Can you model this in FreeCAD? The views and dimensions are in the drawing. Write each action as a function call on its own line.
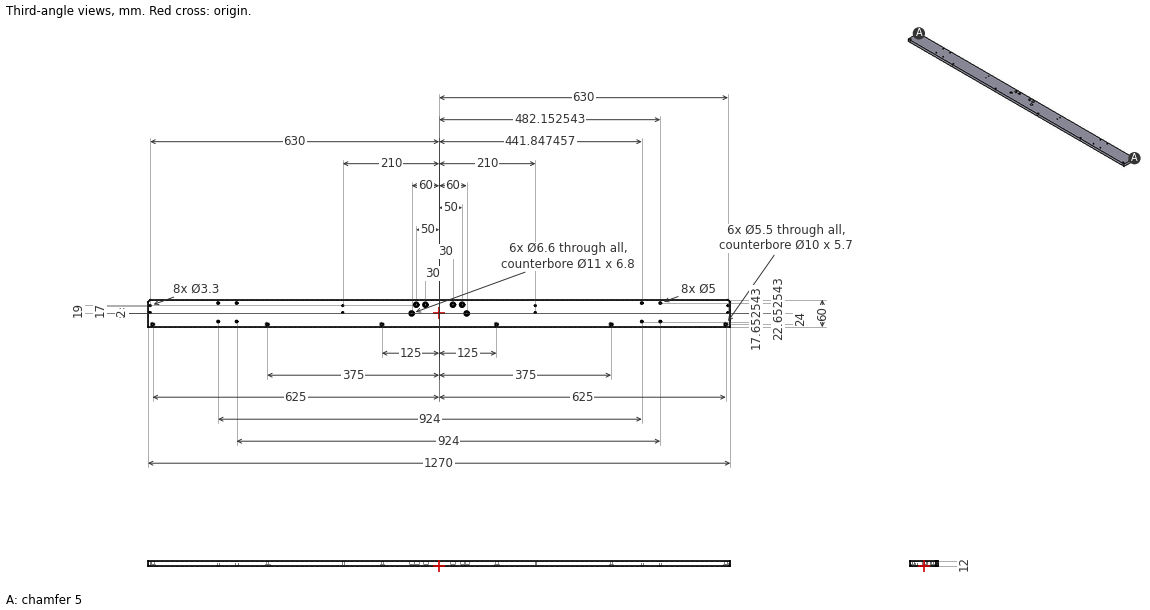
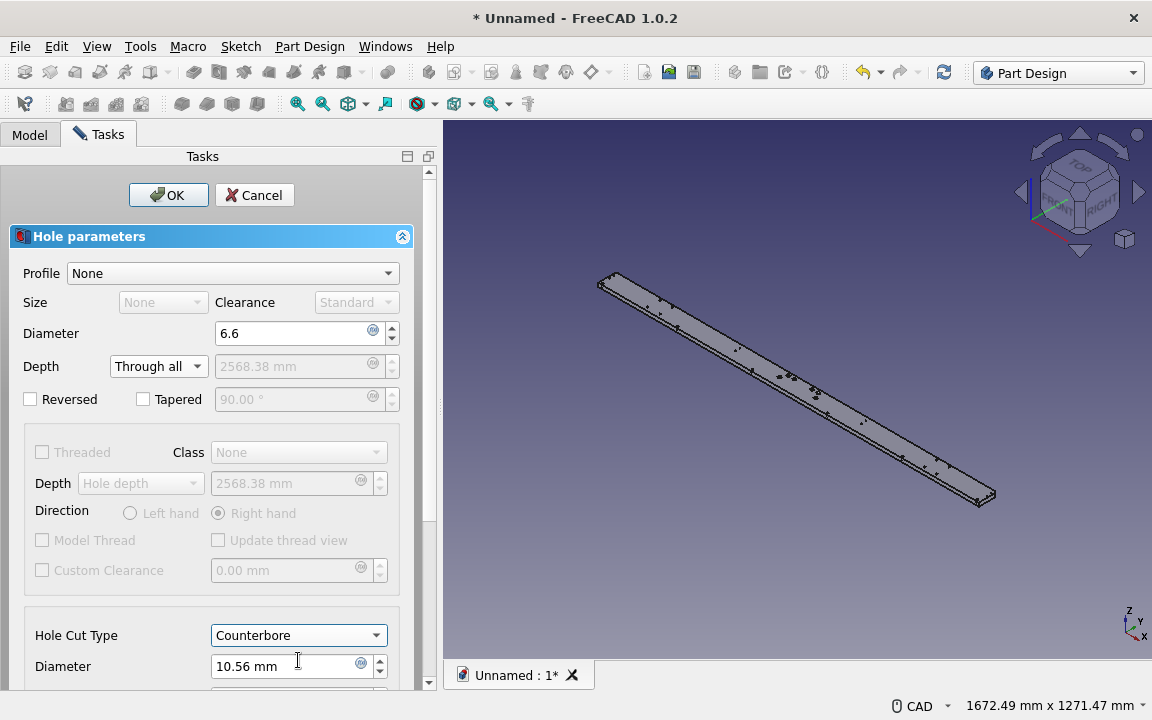
triple_click(292, 666)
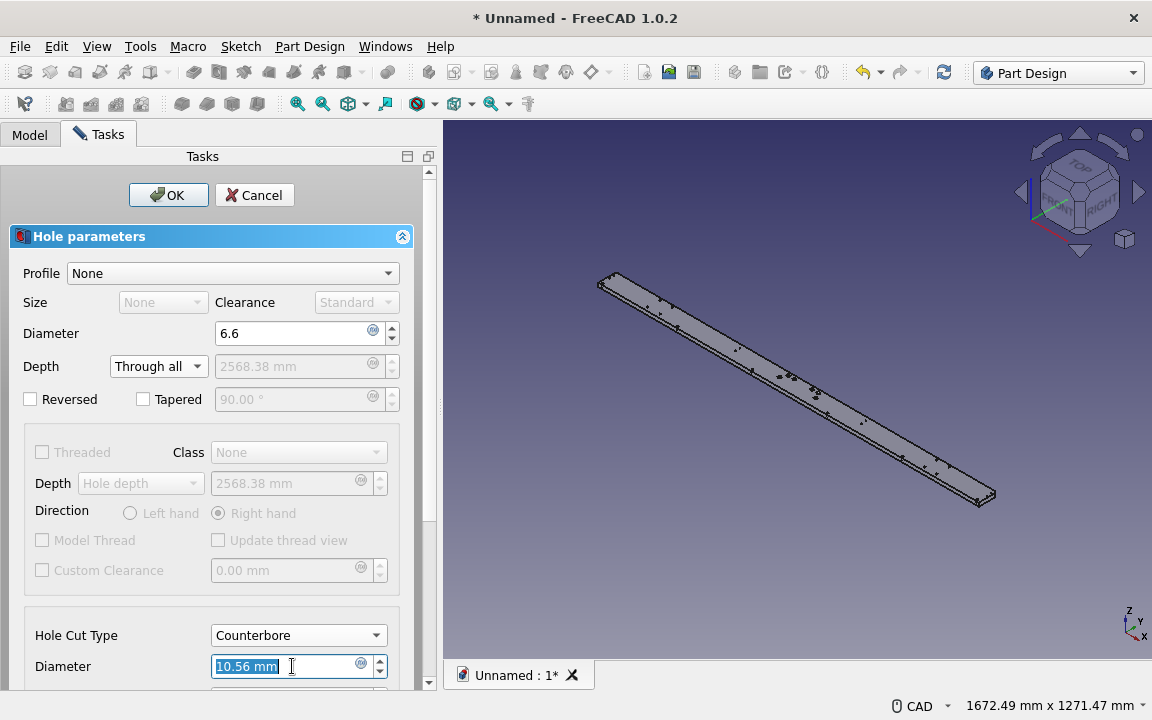
text(11)
key(Tab)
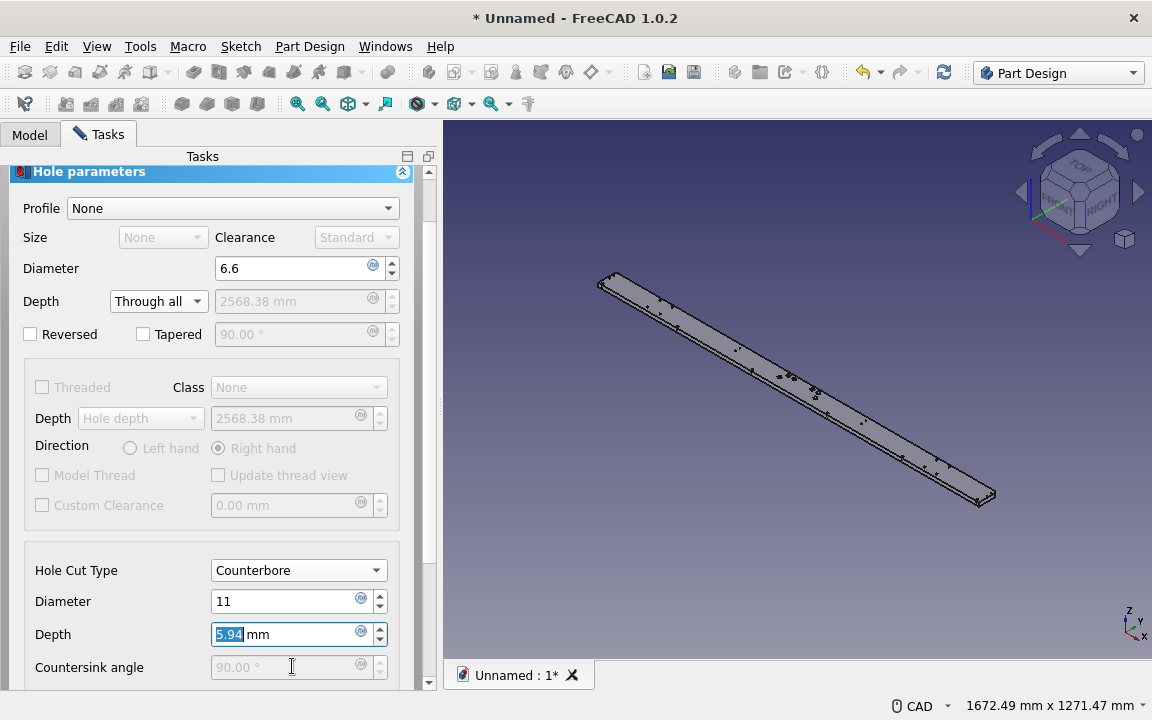
text(6.8)
key(Tab)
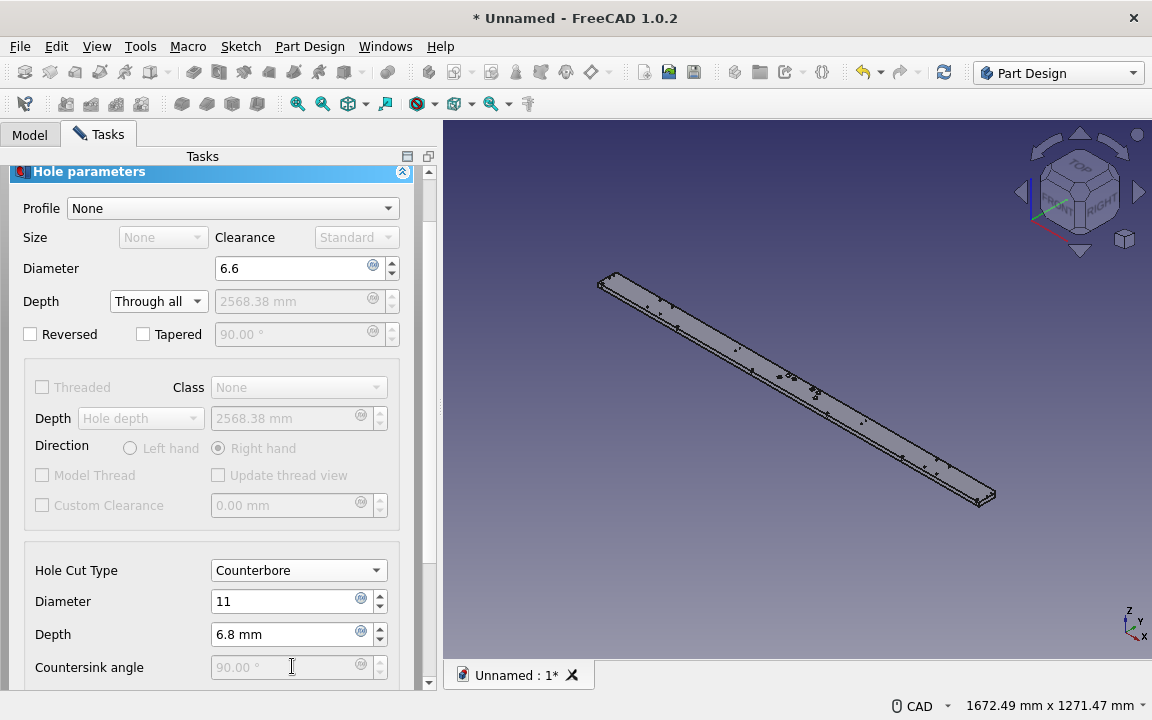
scroll(429, 428, up, 2)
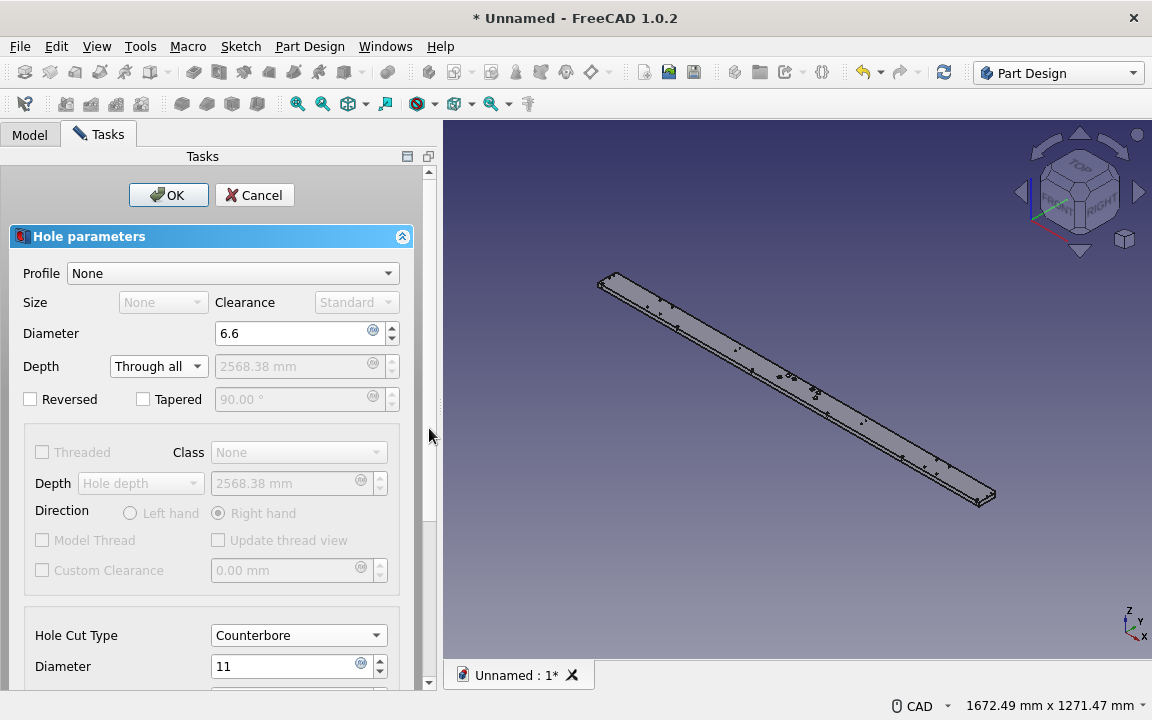
click(169, 195)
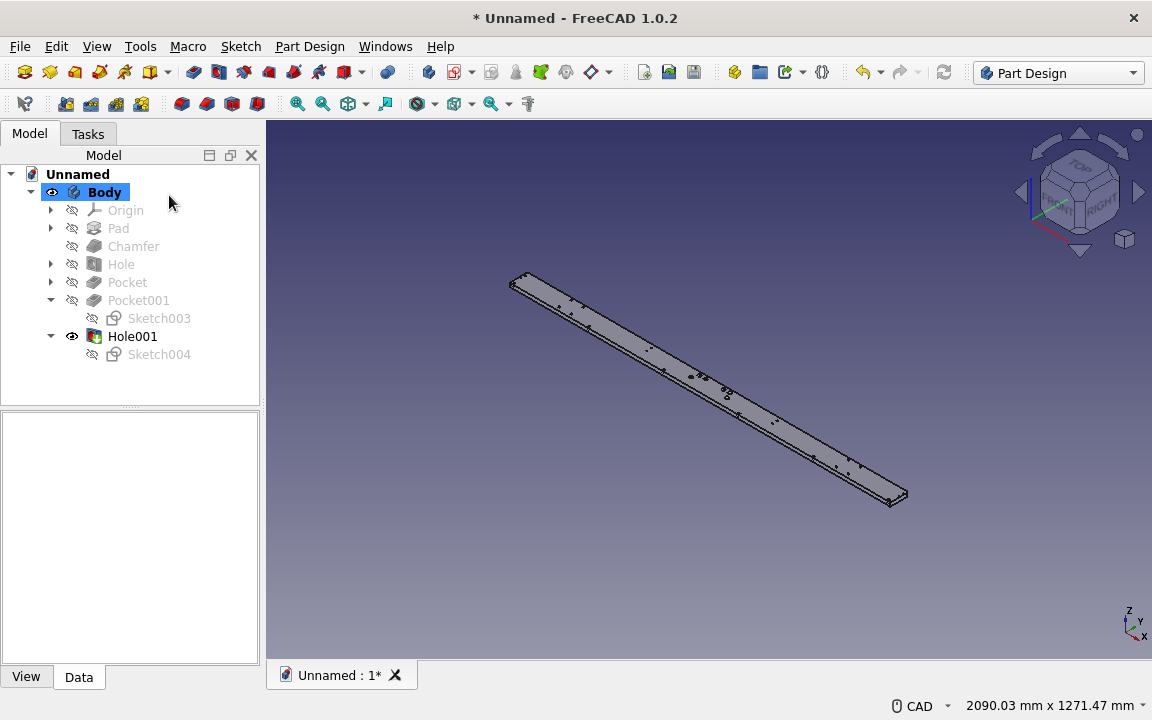
click(298, 104)